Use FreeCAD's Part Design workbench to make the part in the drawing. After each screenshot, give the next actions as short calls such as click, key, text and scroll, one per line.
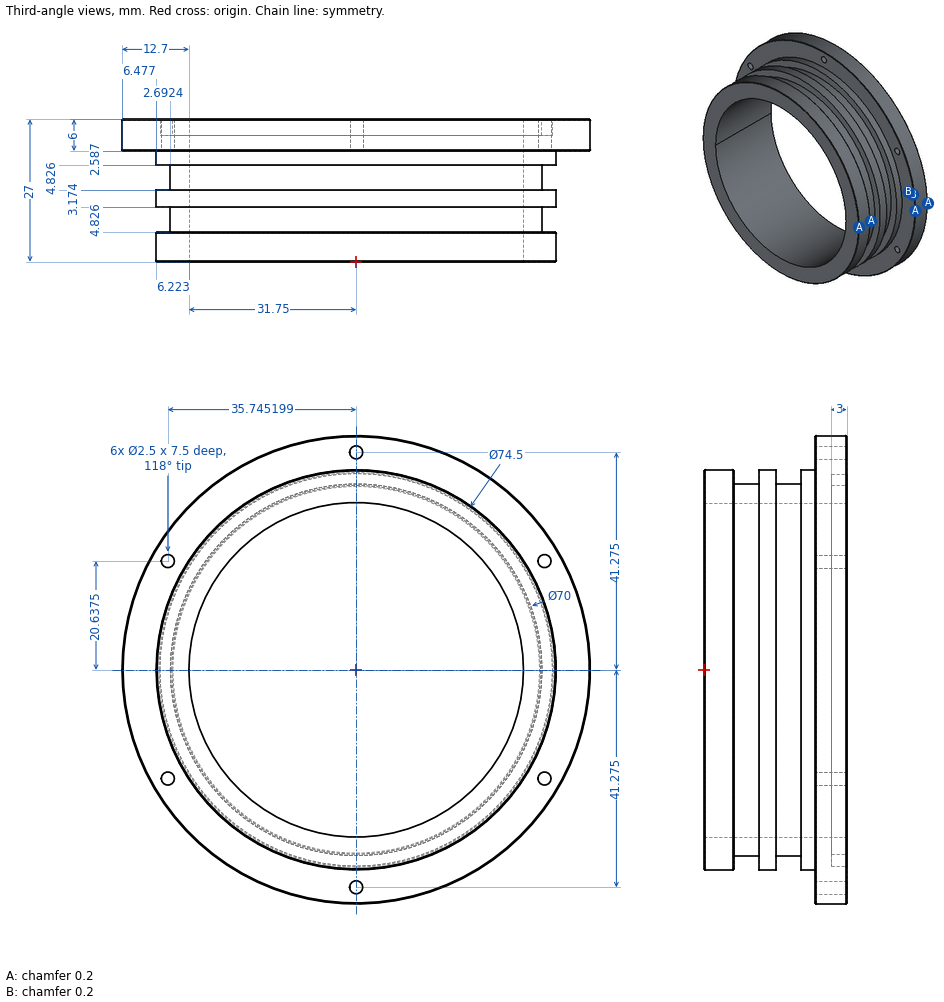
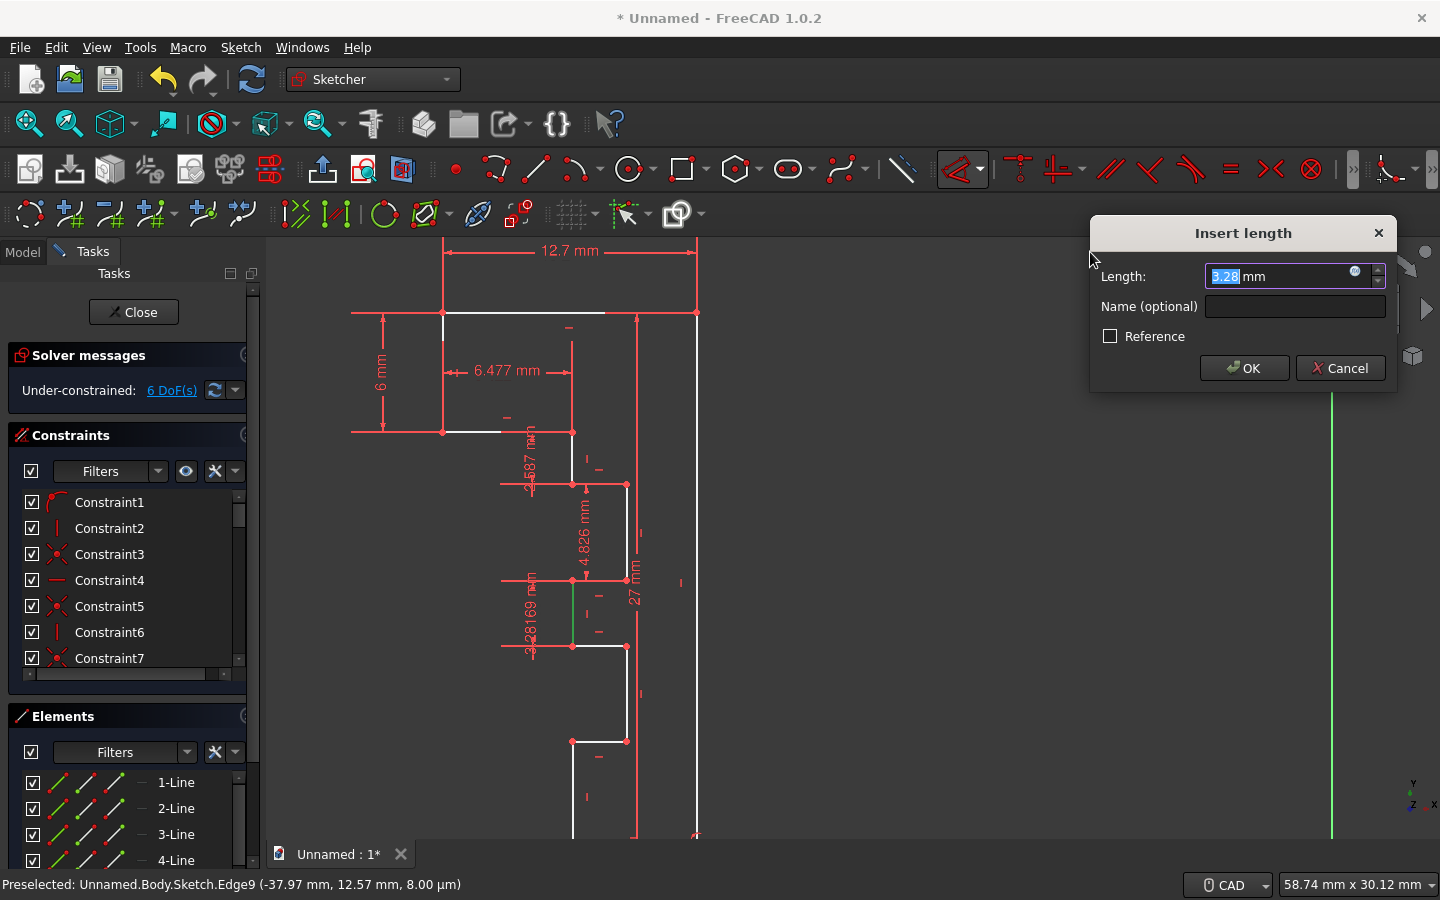
text(3.174)
key(Return)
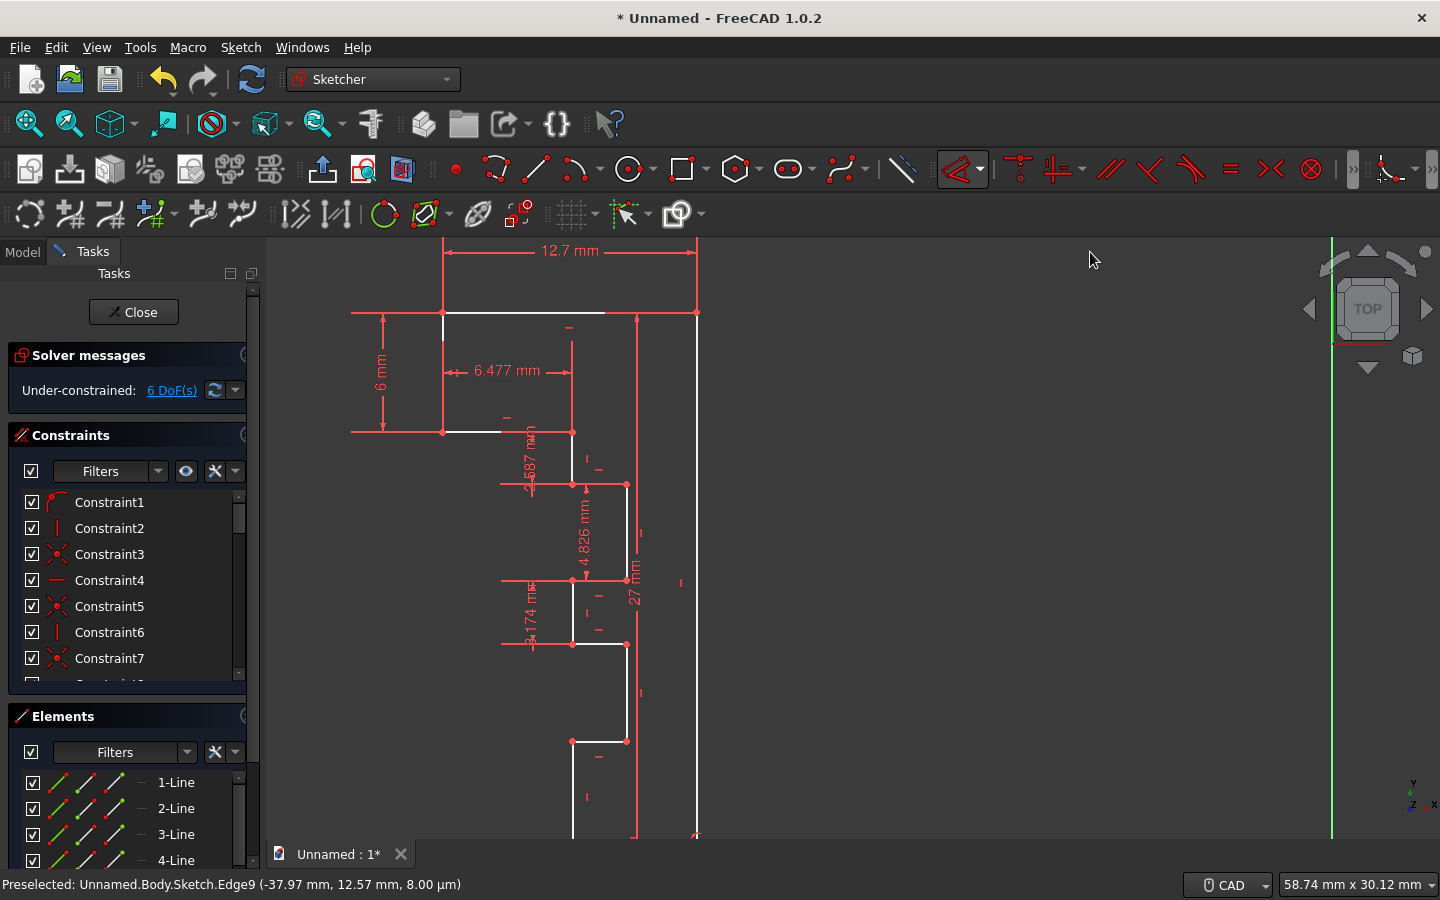
click(627, 673)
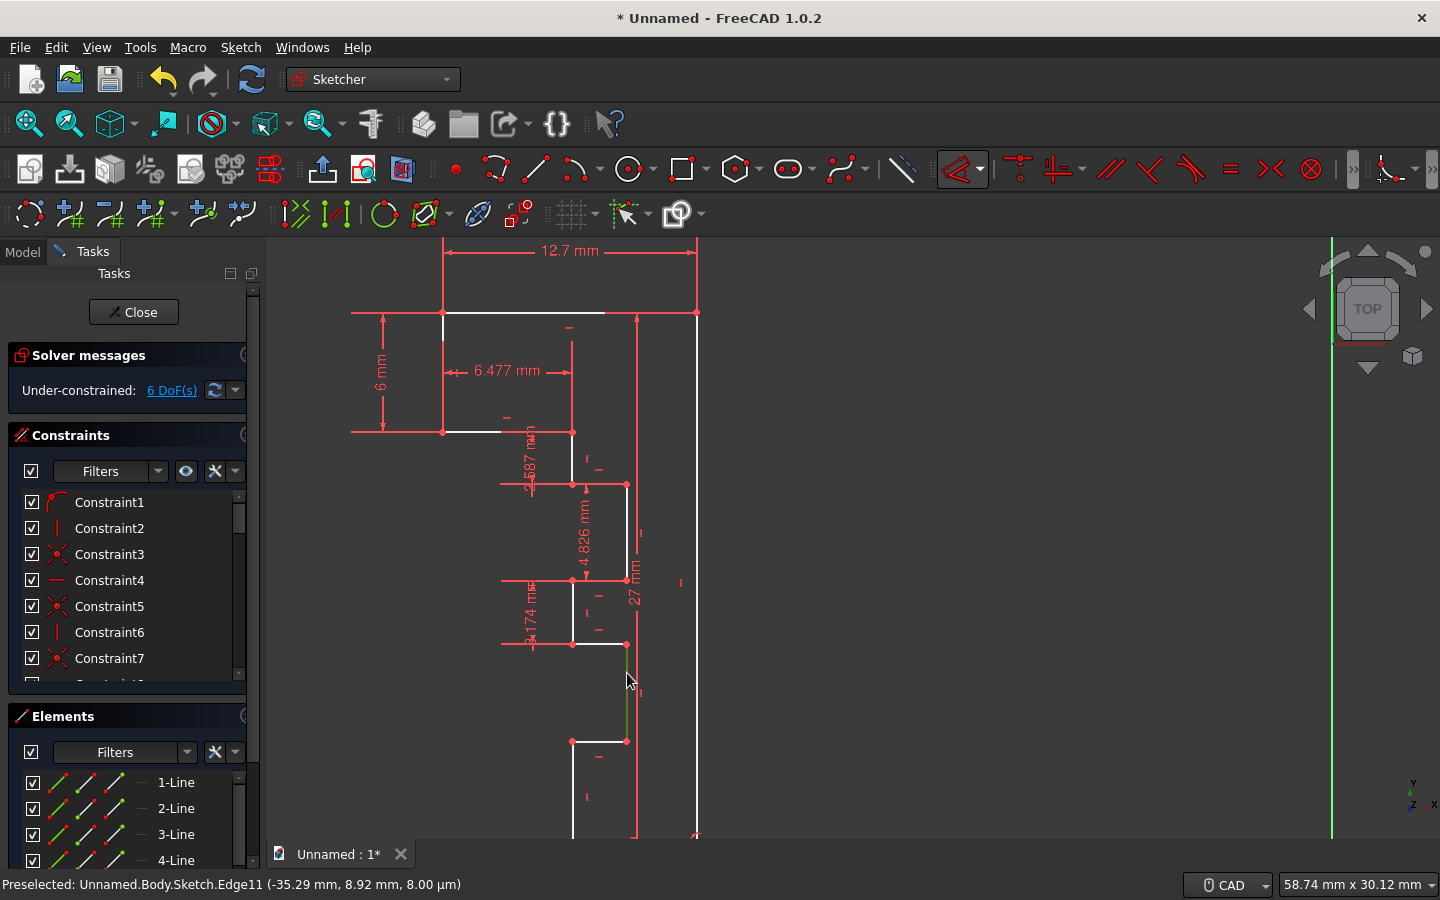
key(i)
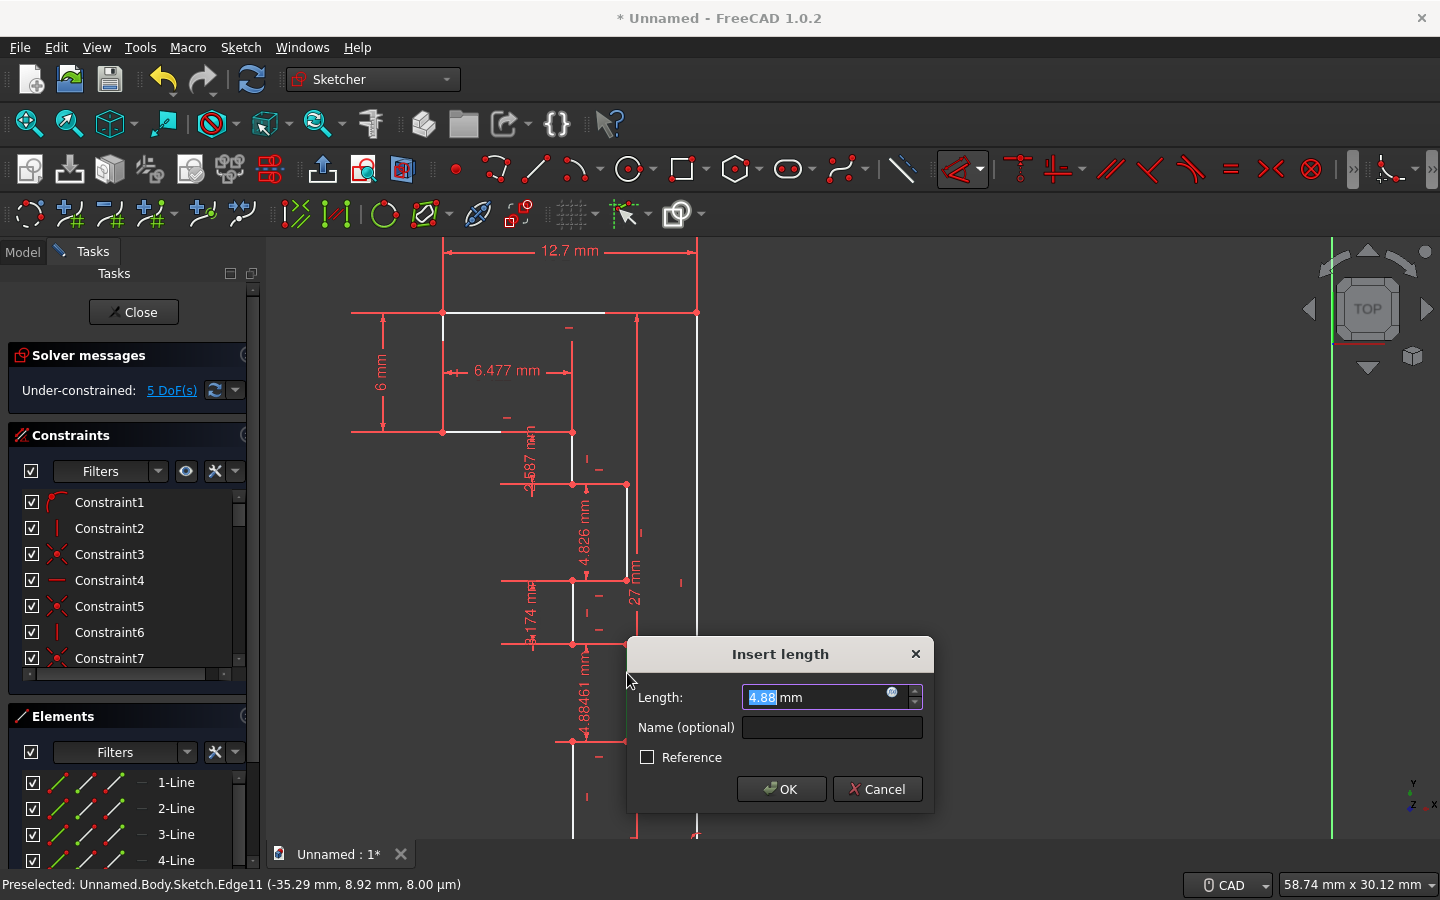
text(4.826)
key(Return)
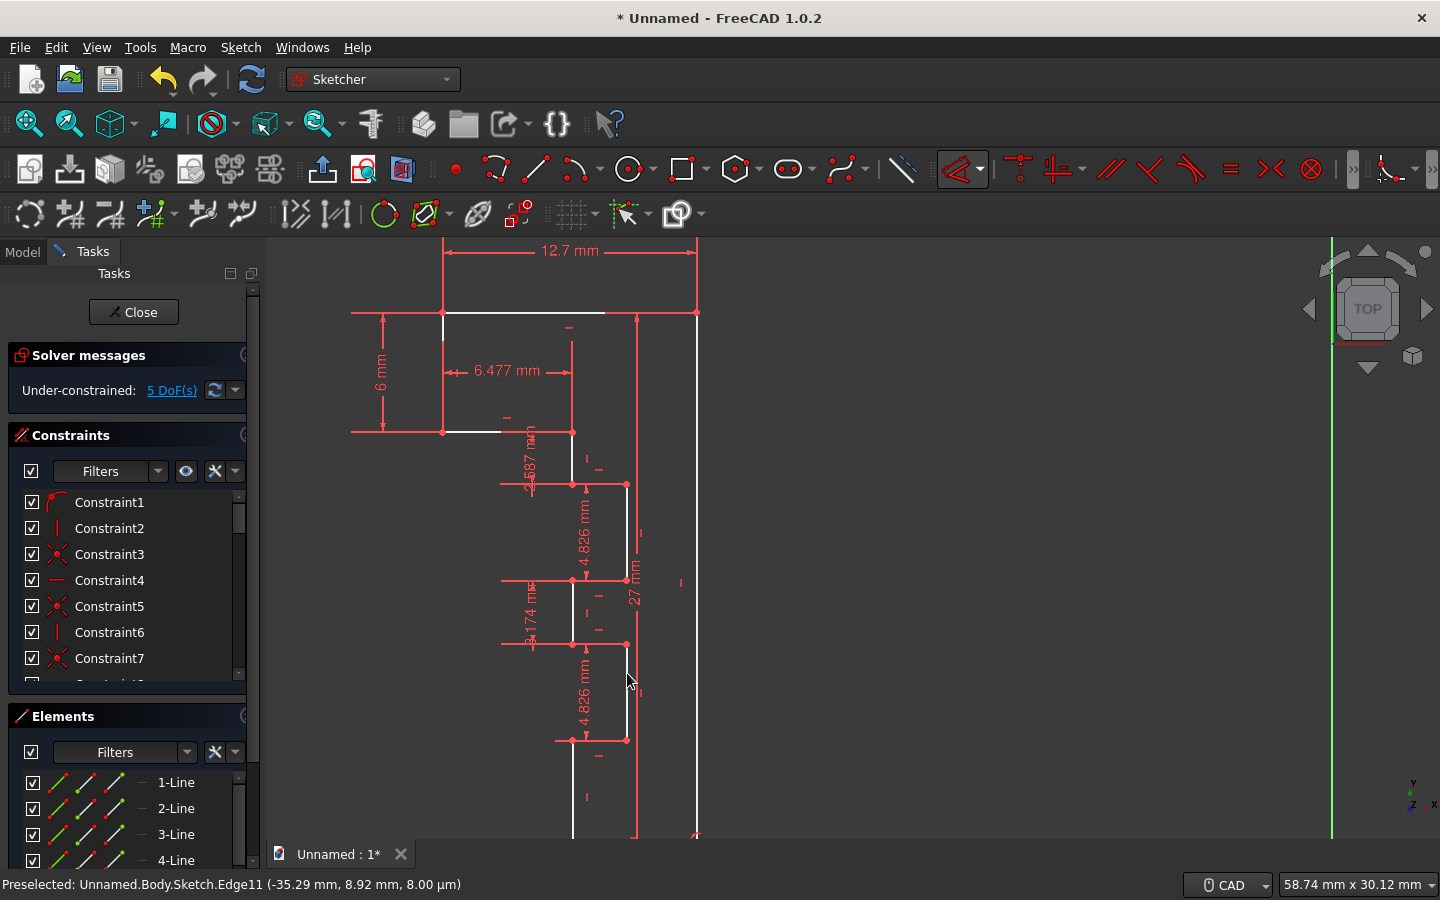
scroll(575, 448, down, 2)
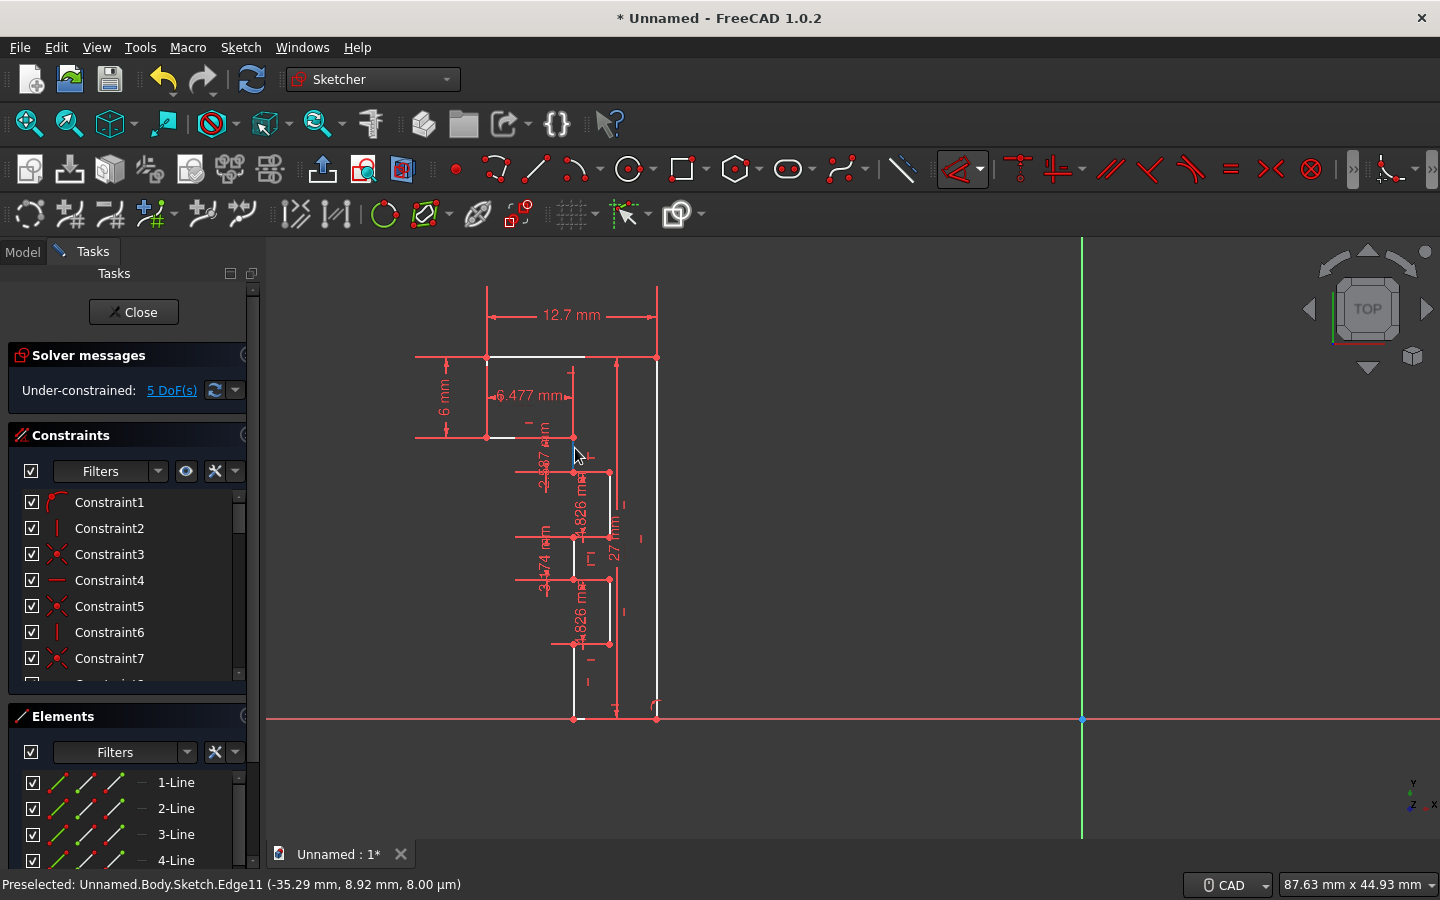
click(599, 719)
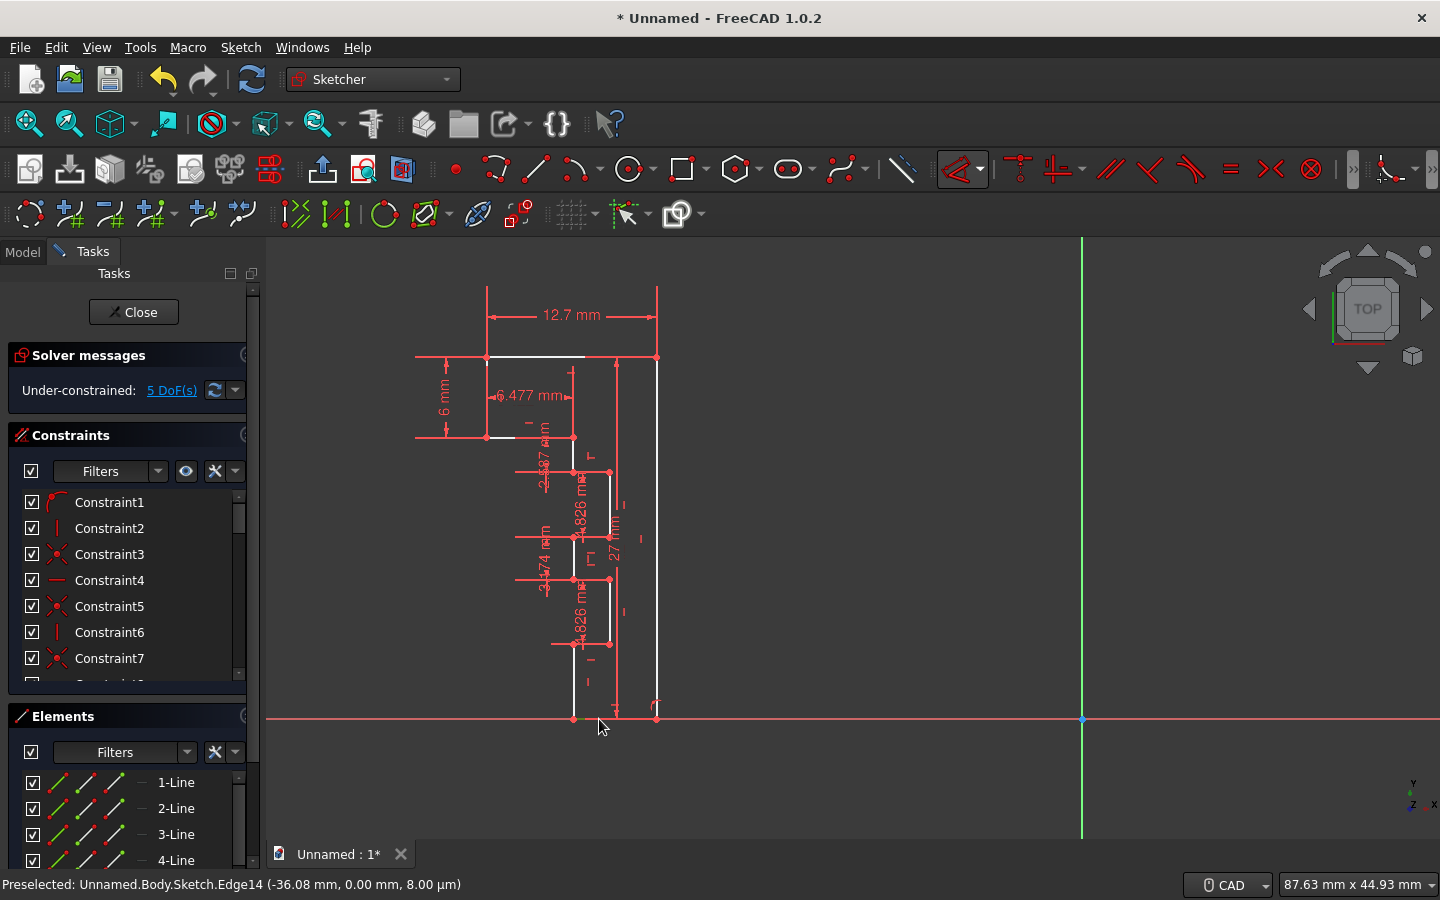
key(l)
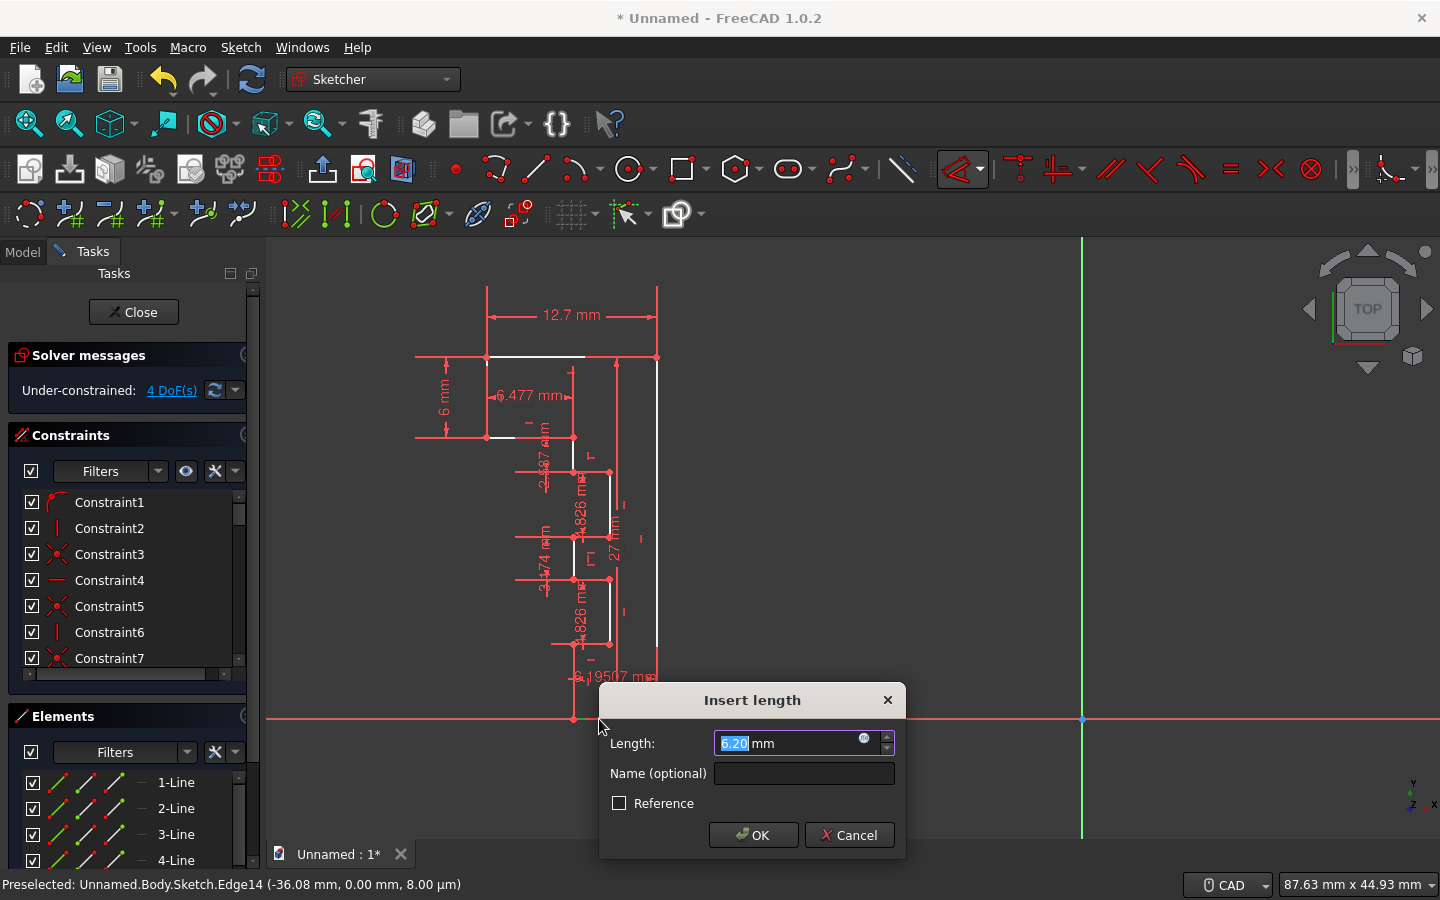
text(6.223)
key(Return)